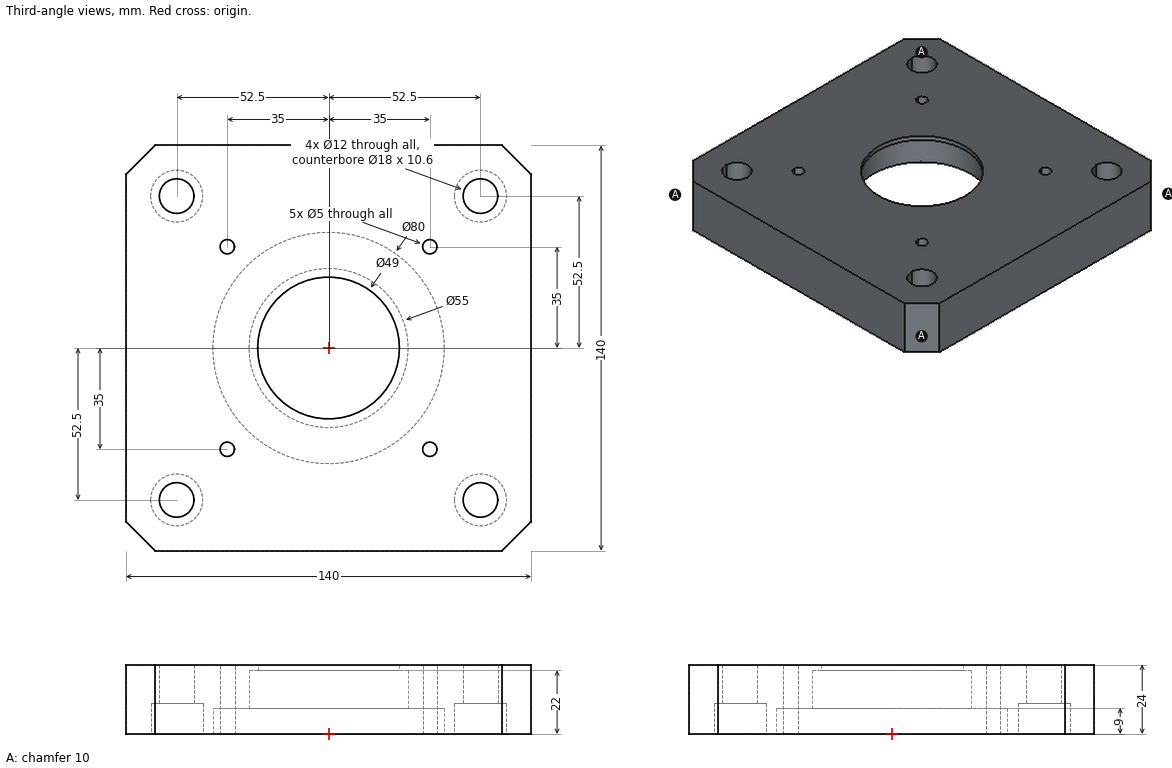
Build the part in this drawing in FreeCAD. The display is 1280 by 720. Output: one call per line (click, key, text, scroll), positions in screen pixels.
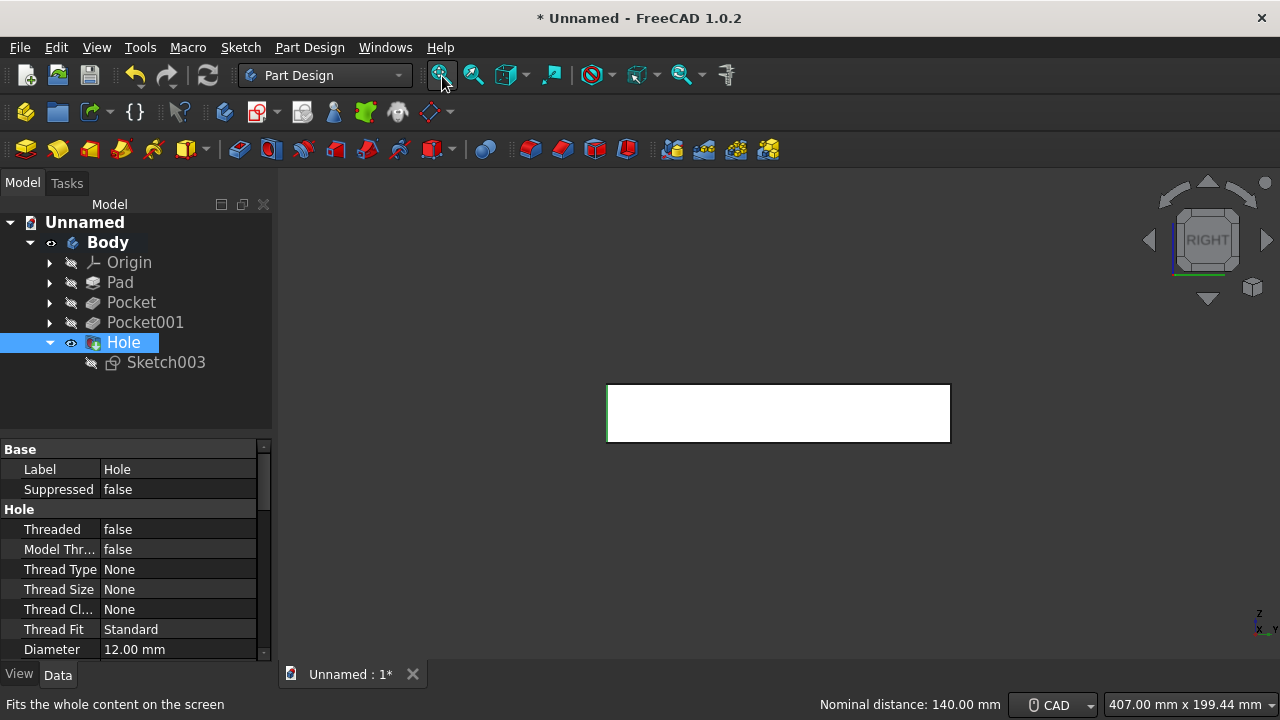
click(951, 412, ctrl)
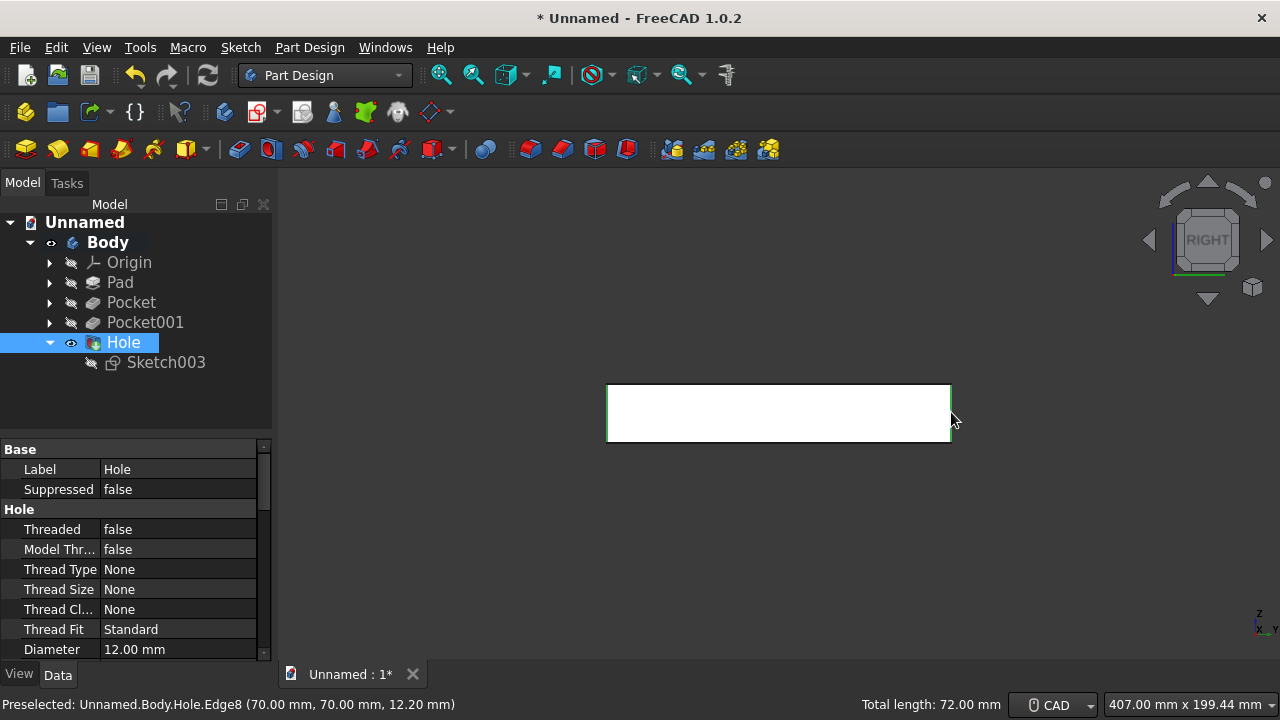
key(5)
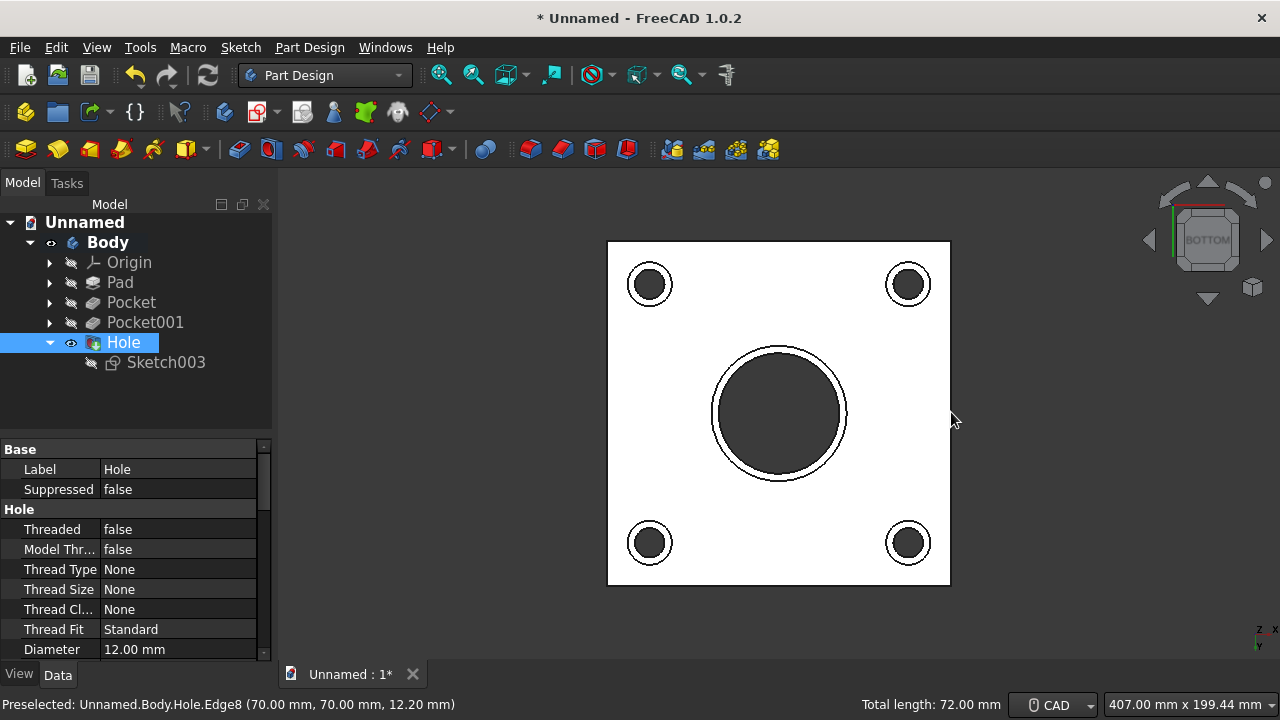
key(4)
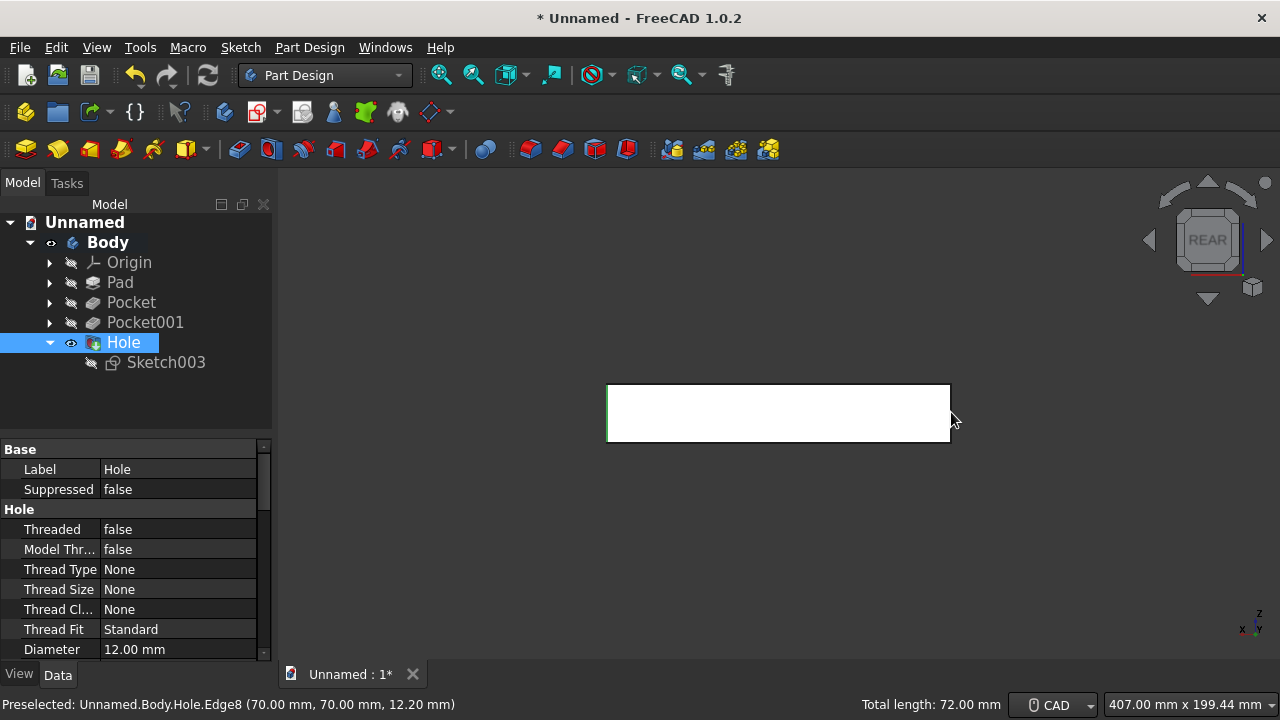
click(442, 76)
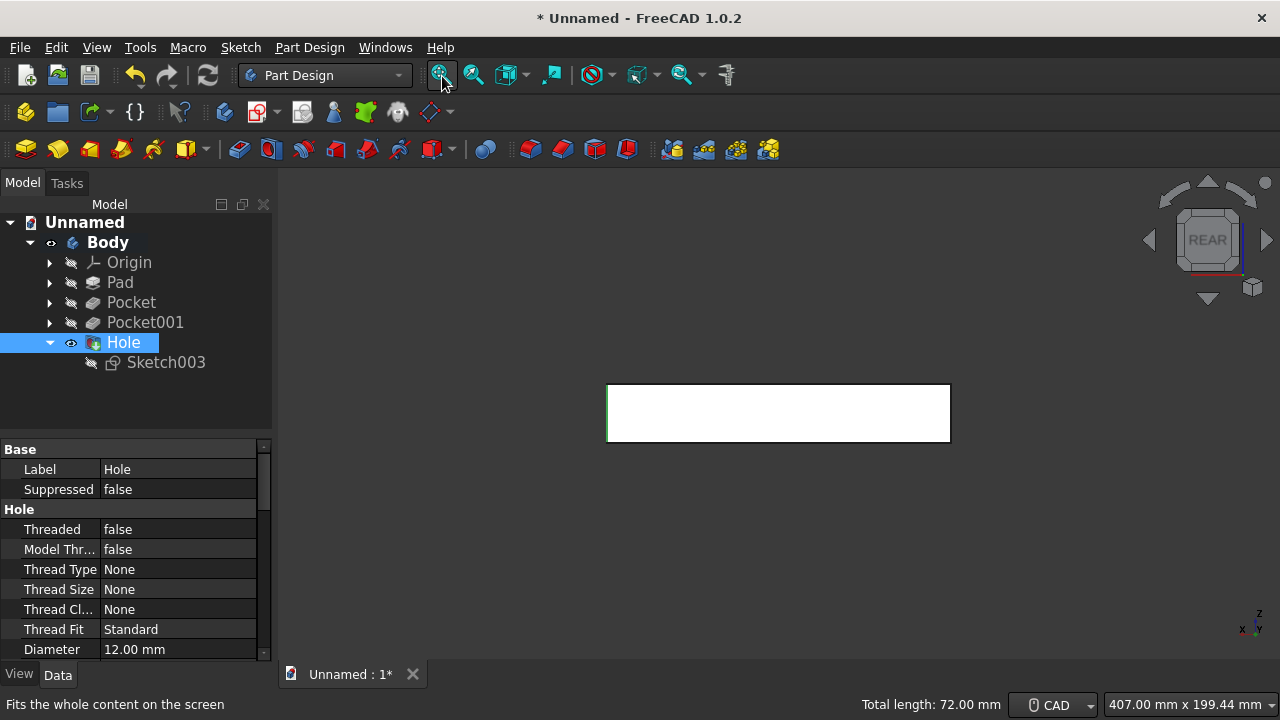
click(951, 413, ctrl)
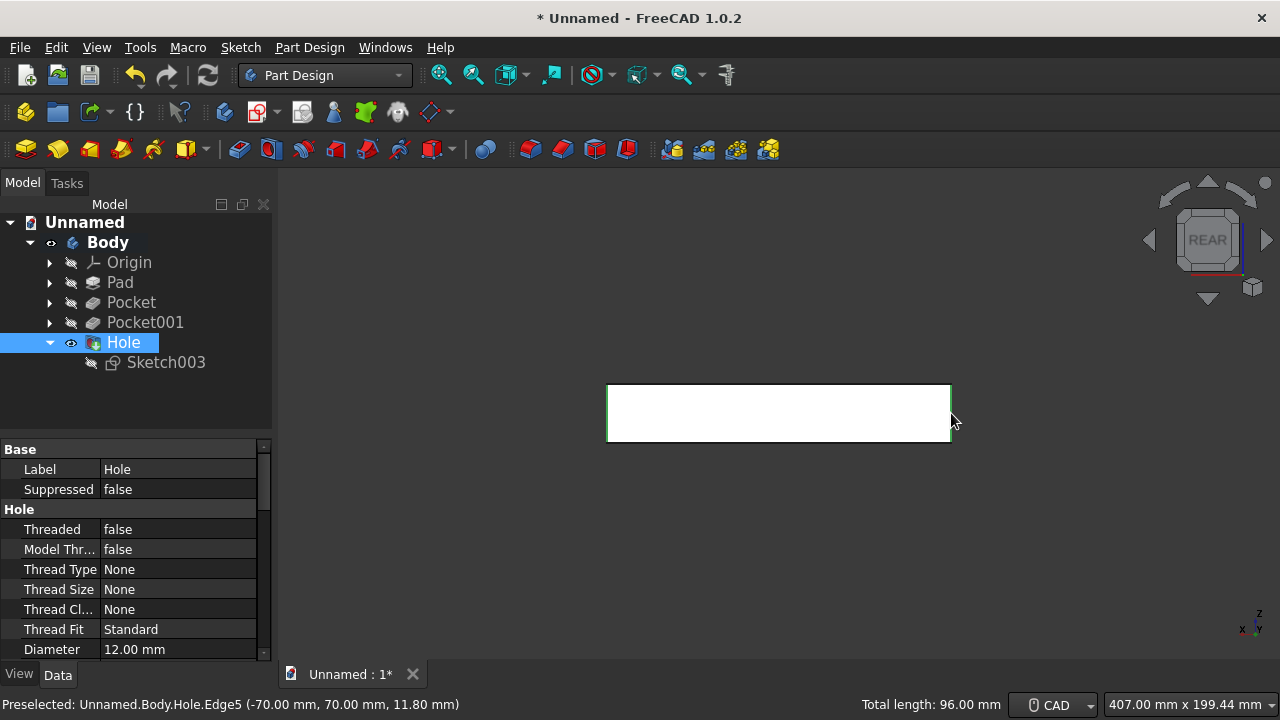
click(564, 150)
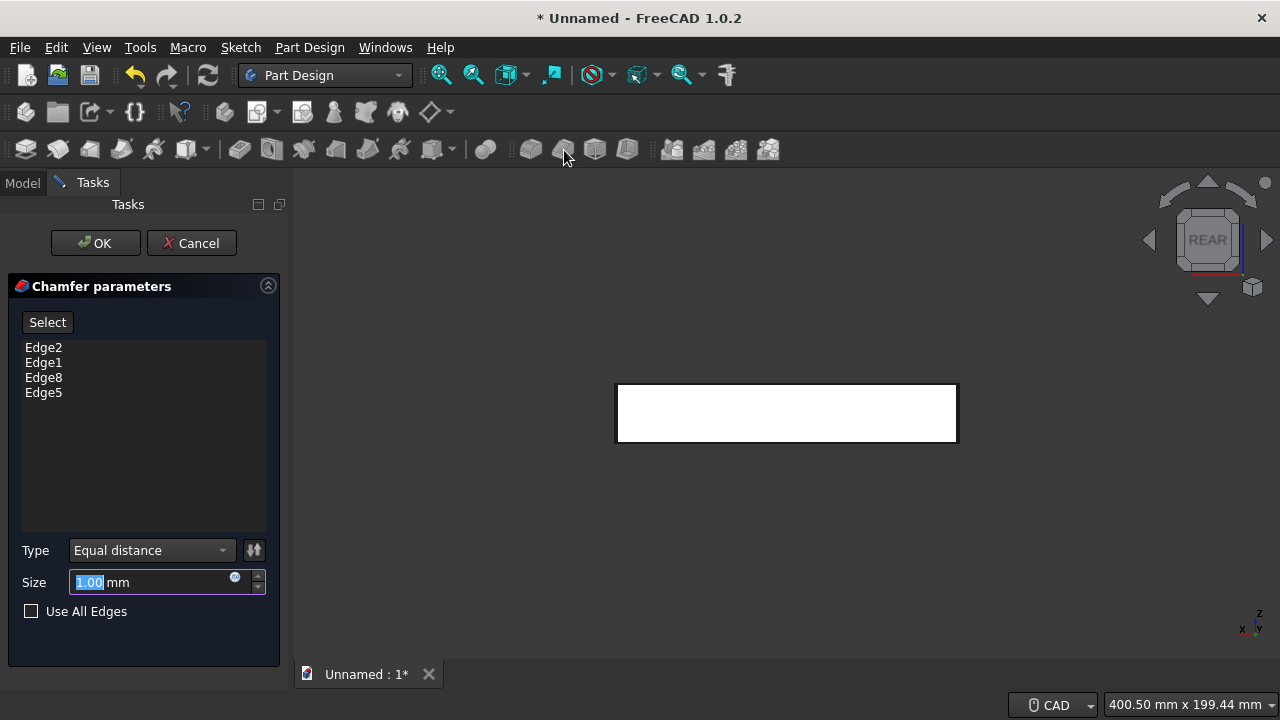
text(10)
key(Tab)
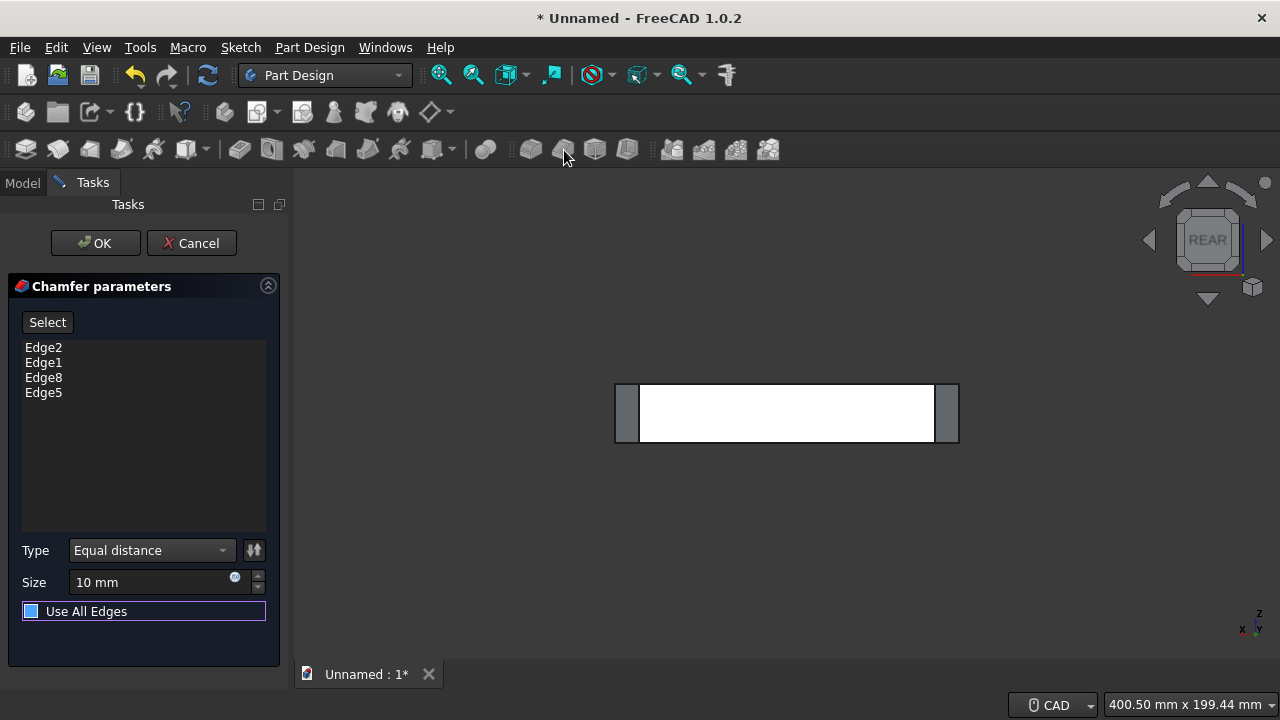
click(96, 243)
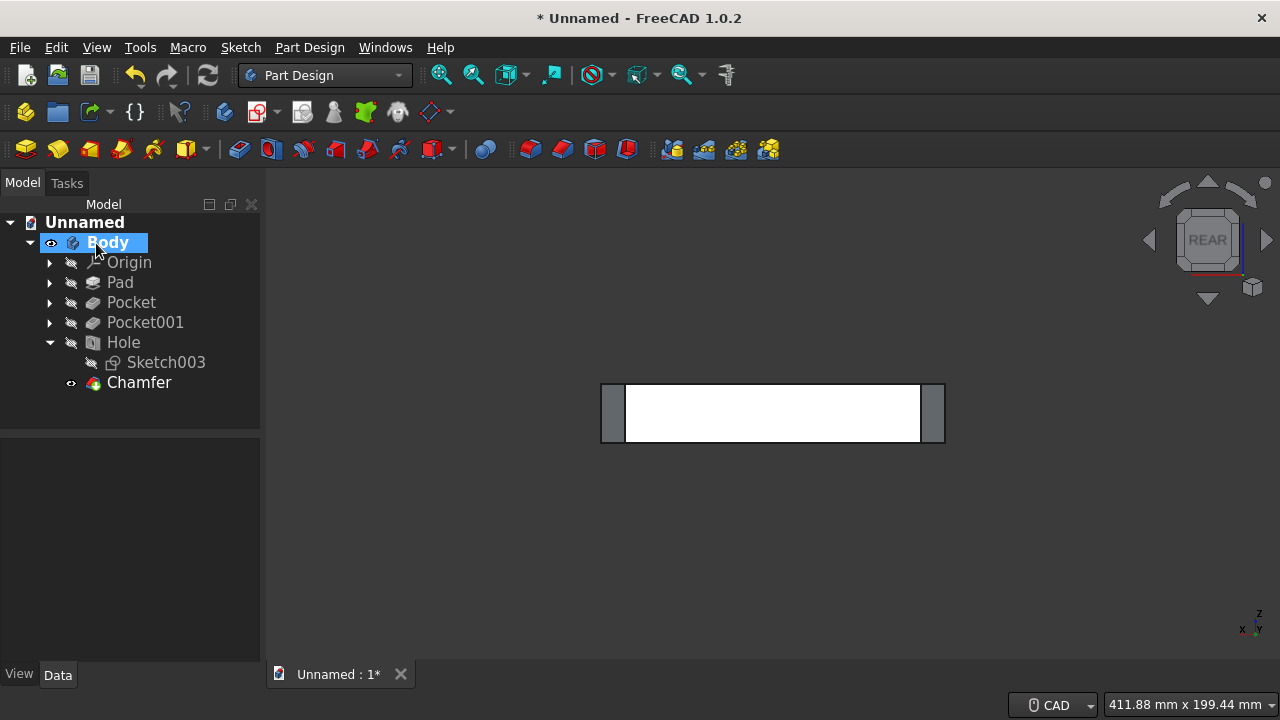
click(442, 76)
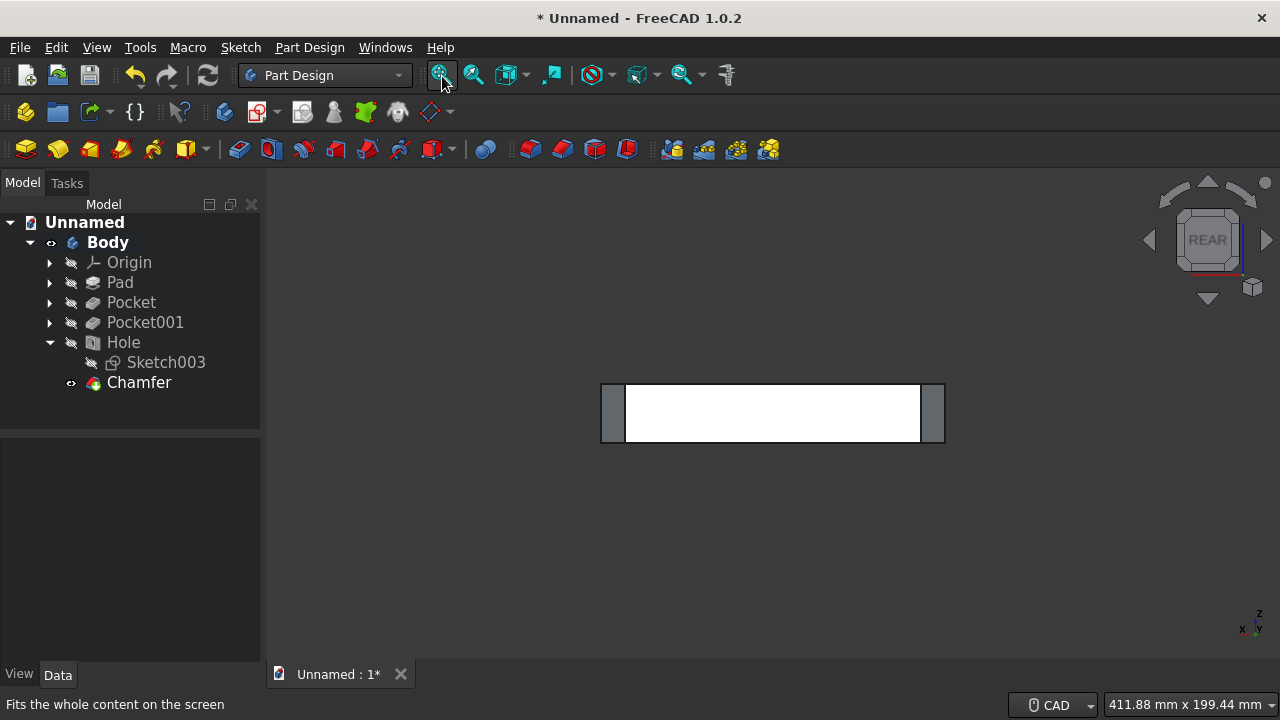
click(258, 112)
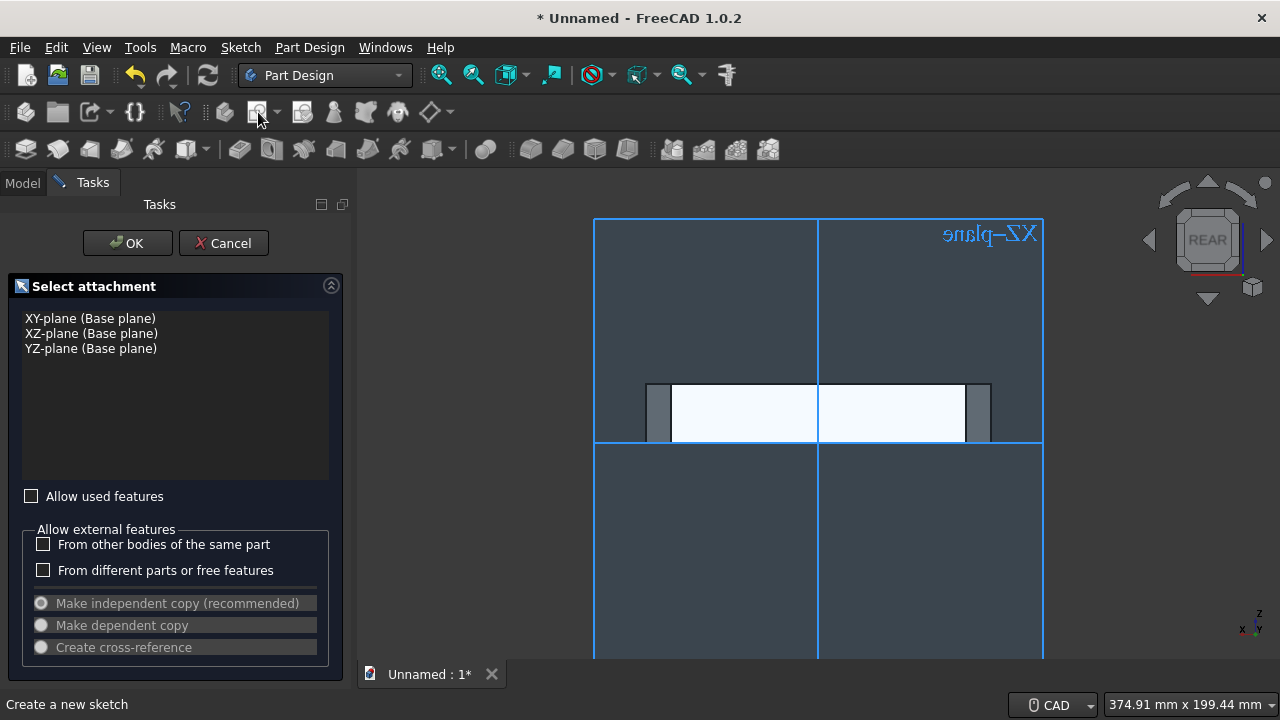
click(82, 318)